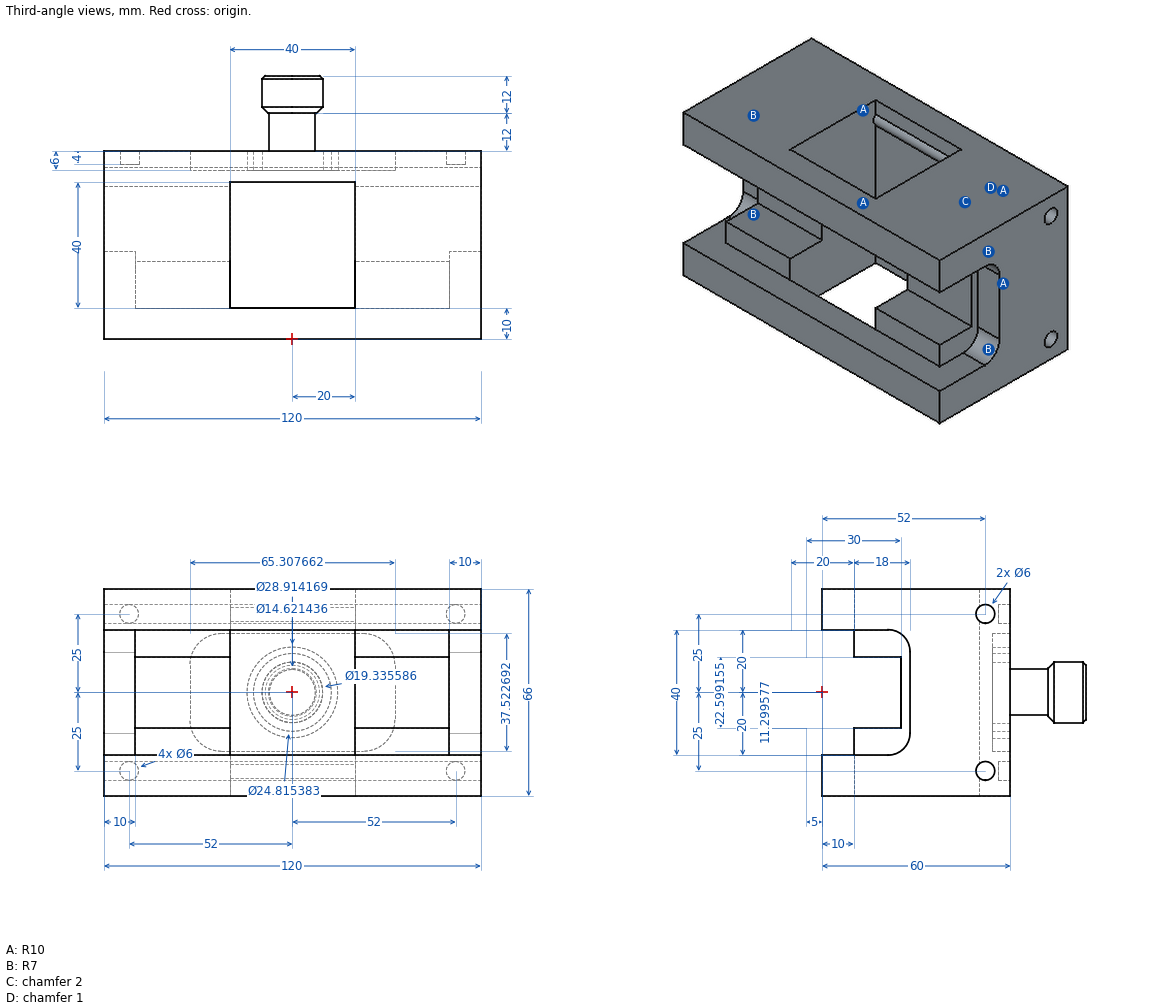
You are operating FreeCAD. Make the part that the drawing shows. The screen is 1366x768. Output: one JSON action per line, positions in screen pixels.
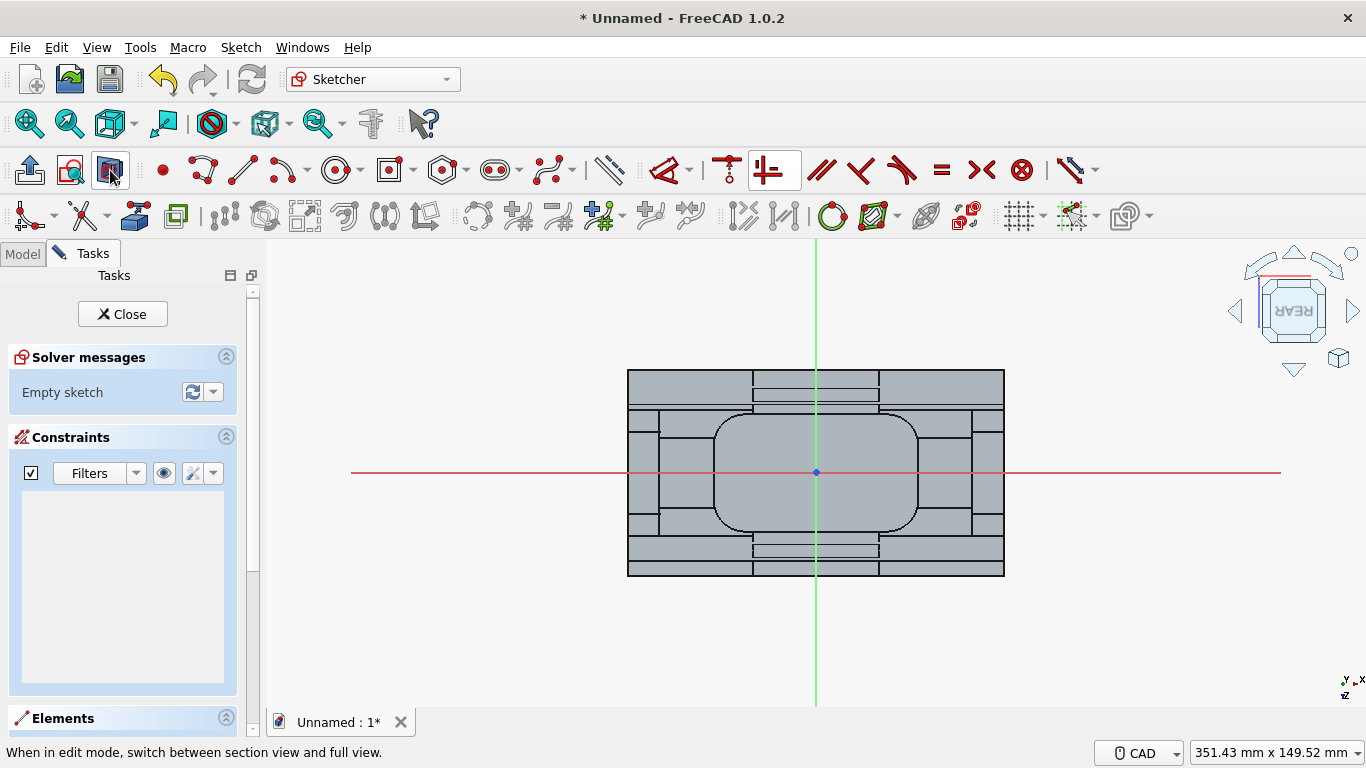
{"action": "scroll", "coordinate": [846, 473], "scroll_direction": "up", "scroll_amount": 6}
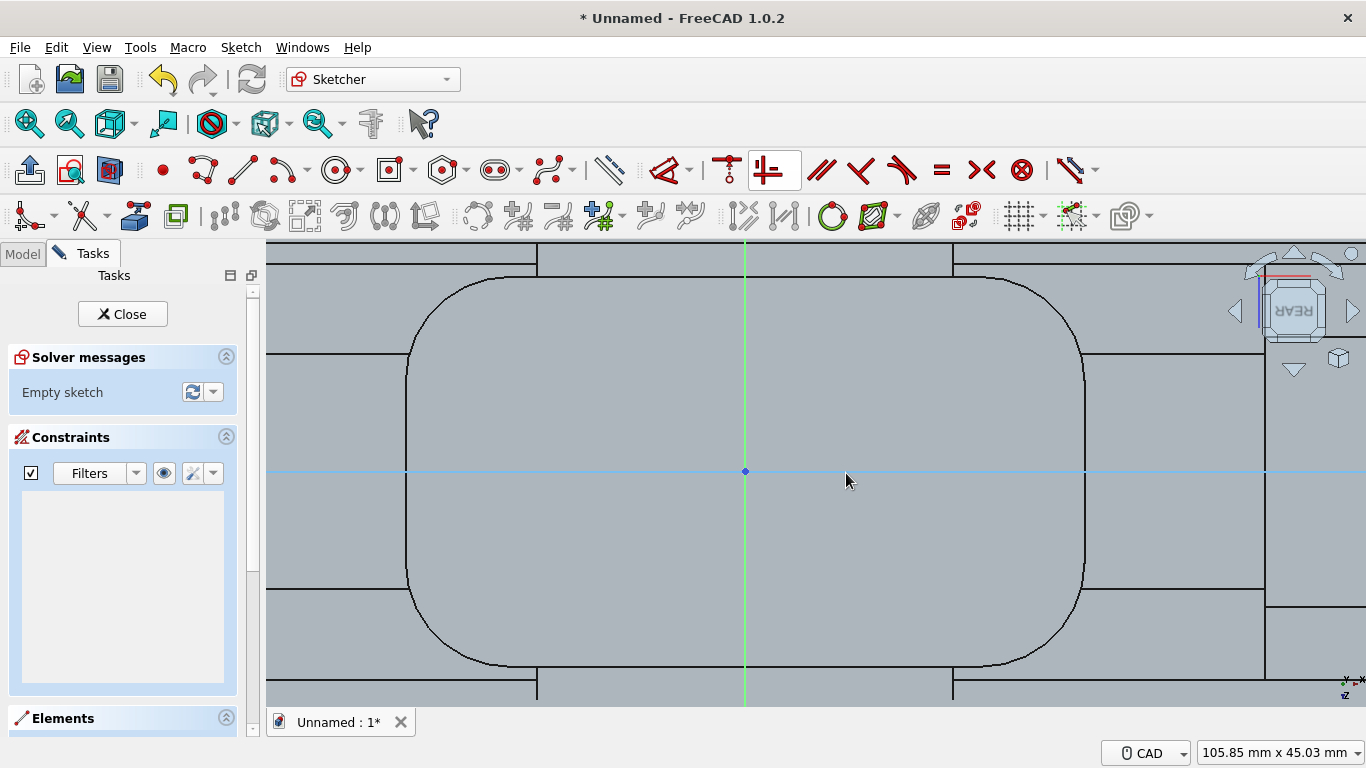
{"action": "left_click", "coordinate": [336, 170]}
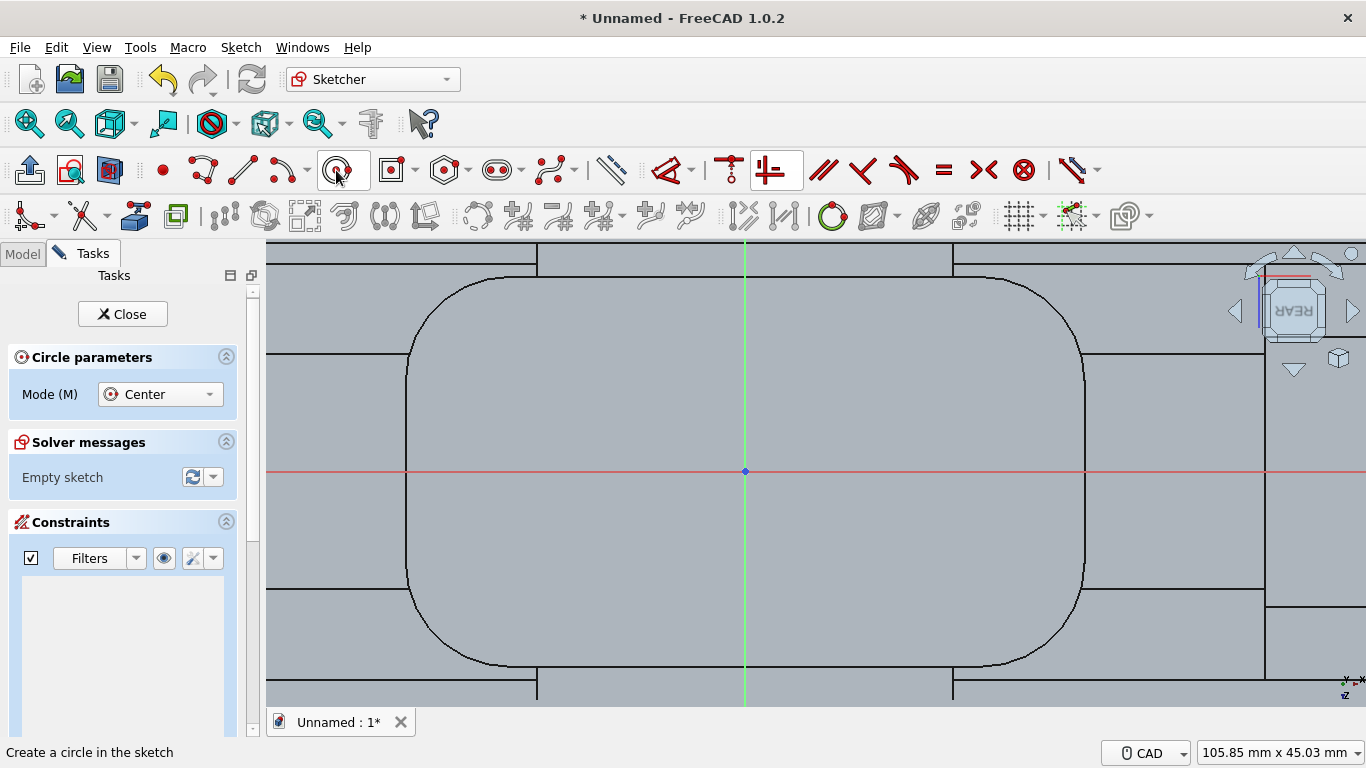
{"action": "left_click", "coordinate": [745, 472]}
{"action": "mouse_move", "coordinate": [851, 366]}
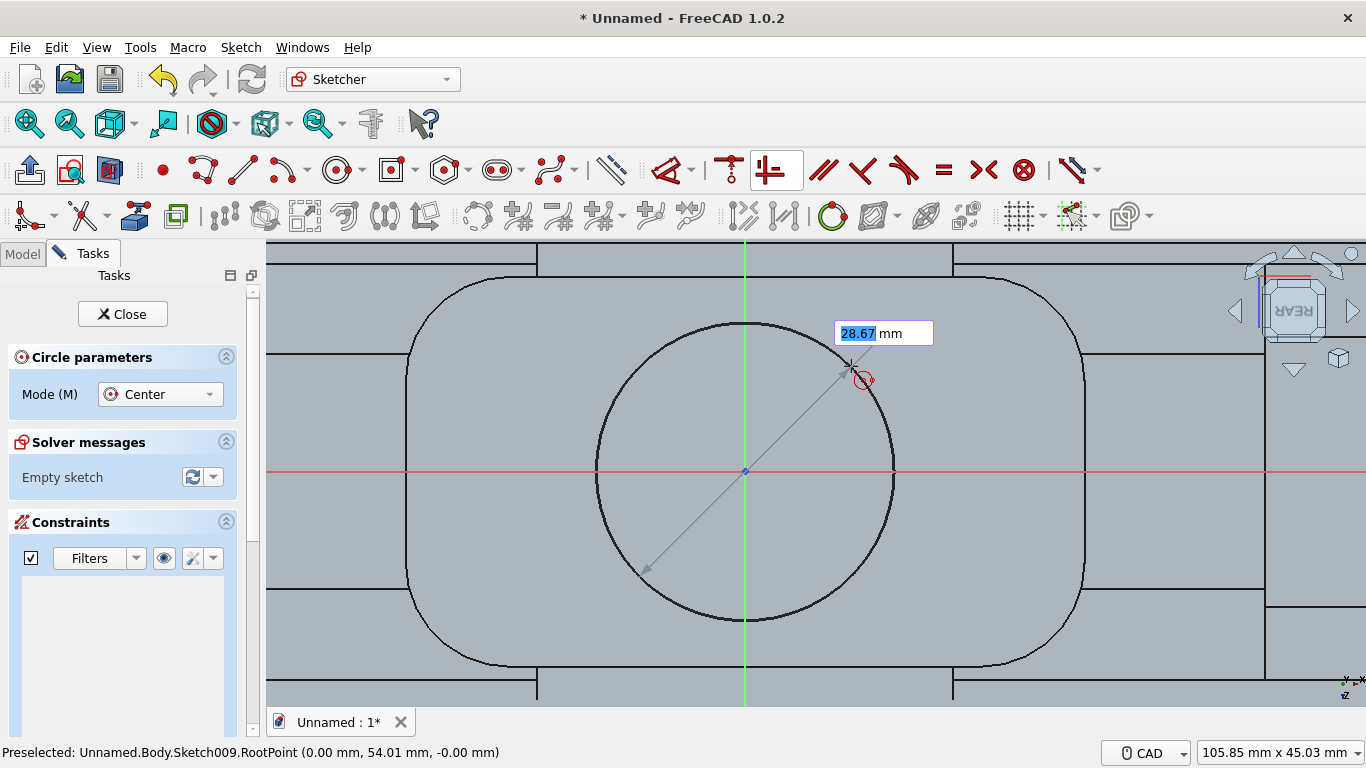
{"action": "type", "text": "28.914169"}
{"action": "key", "text": "Return"}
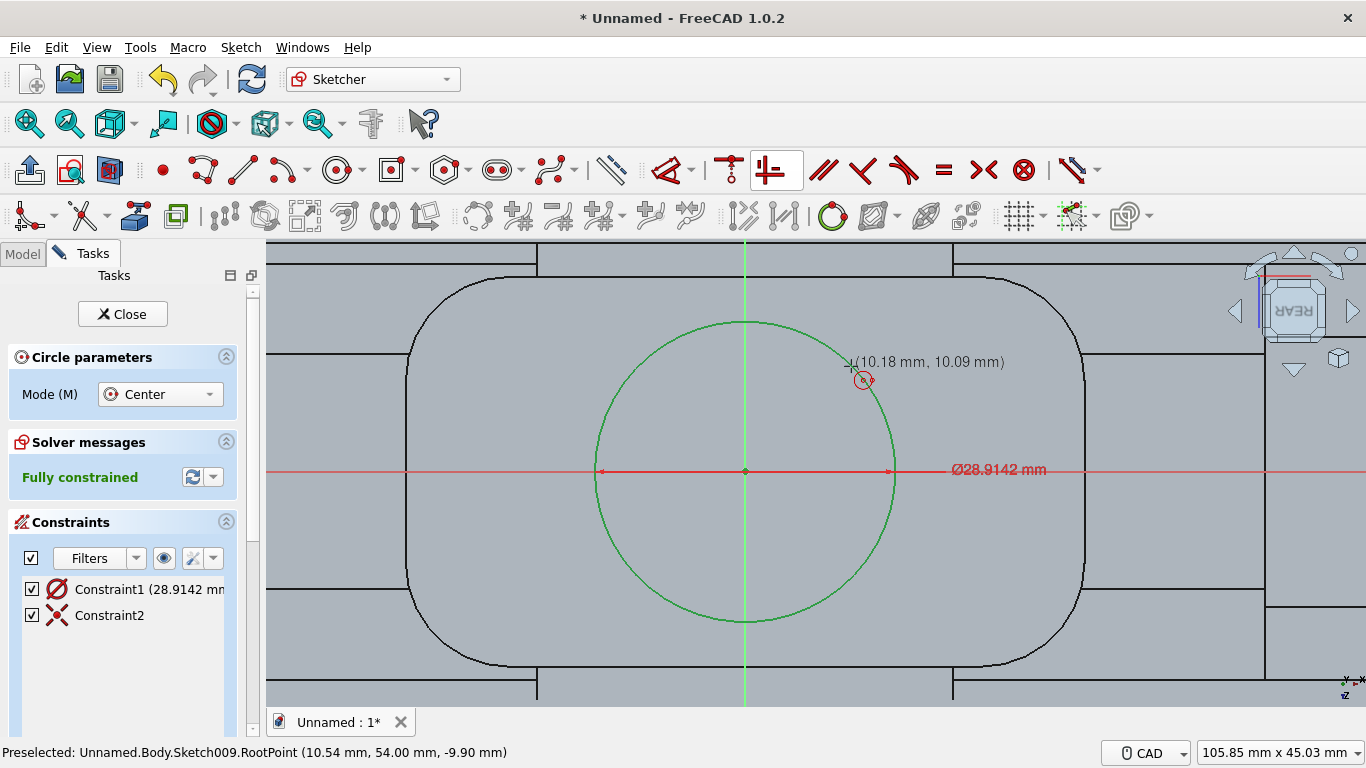
{"action": "left_click", "coordinate": [745, 472]}
{"action": "mouse_move", "coordinate": [836, 381]}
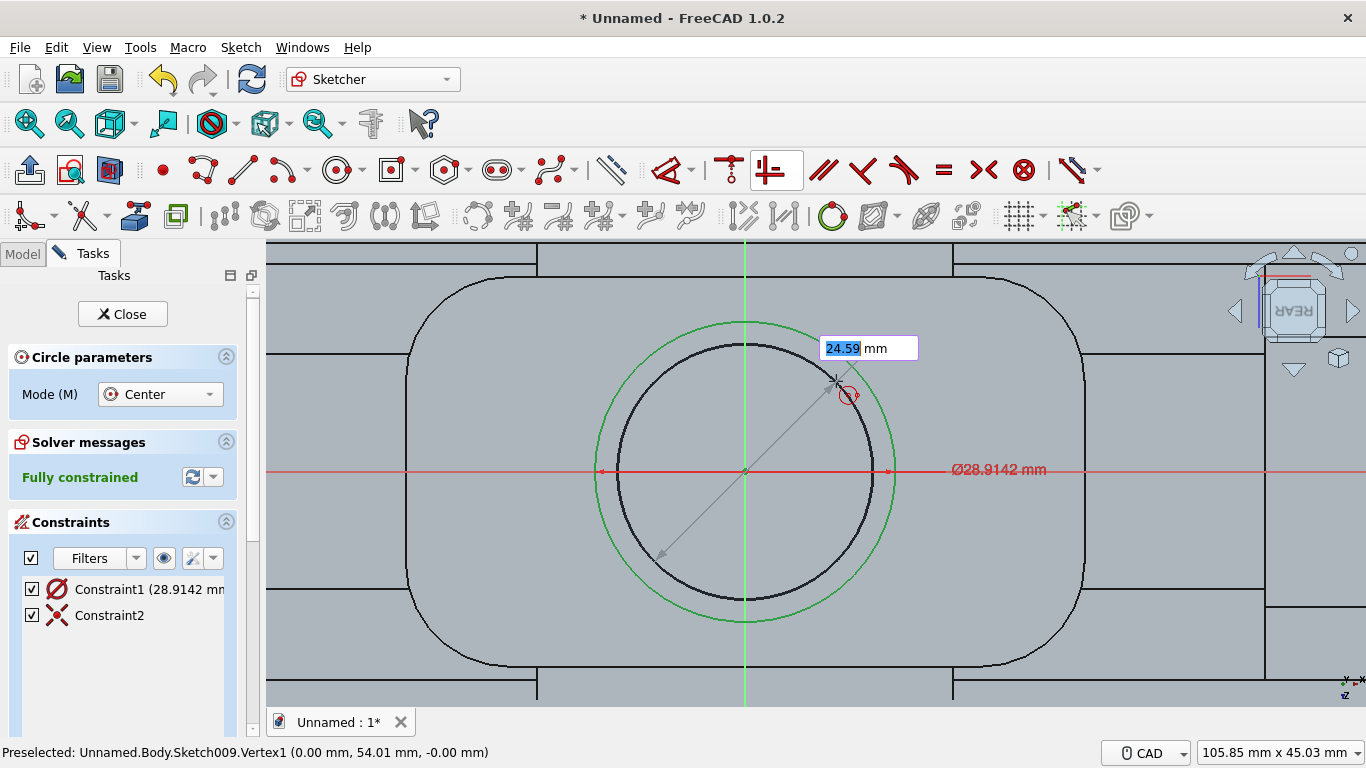
{"action": "type", "text": "24.815383"}
{"action": "key", "text": "Return"}
{"action": "key", "text": "Escape"}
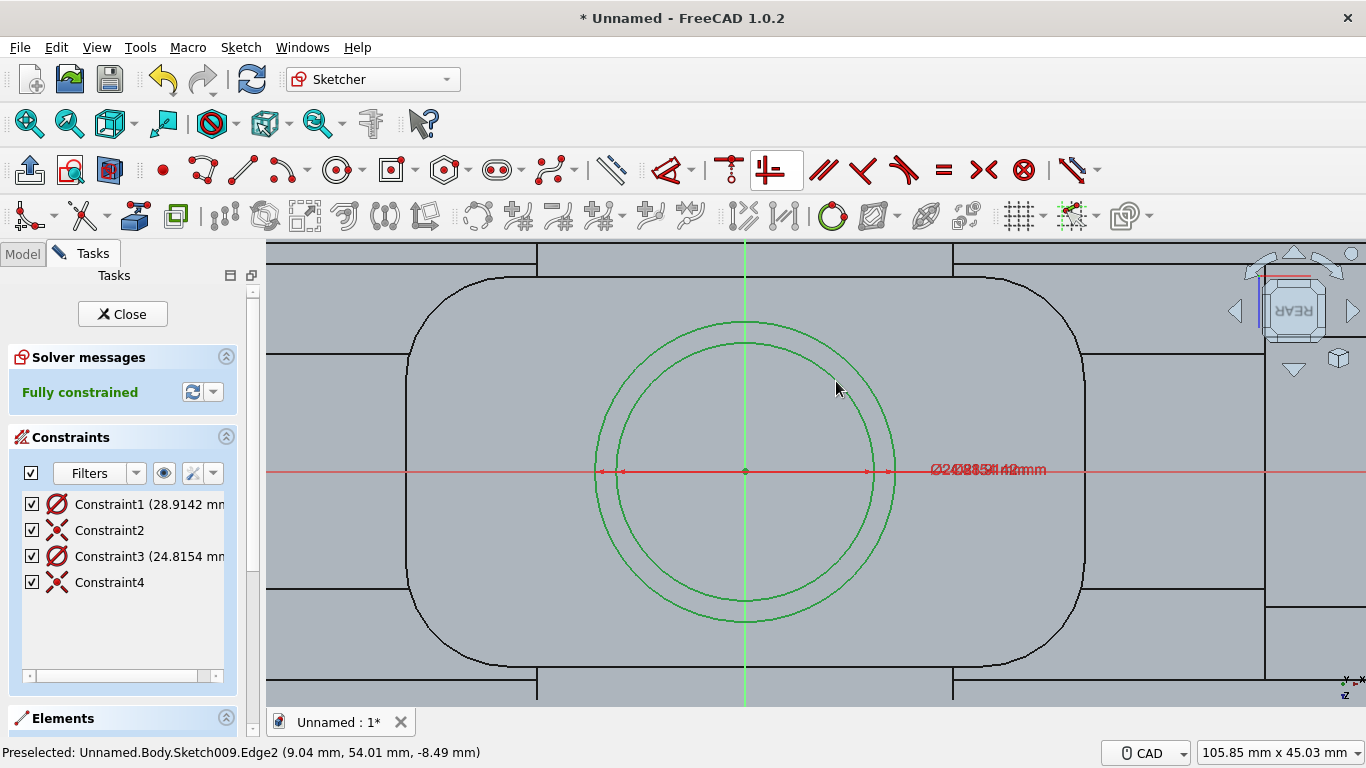
{"action": "left_click", "coordinate": [123, 314]}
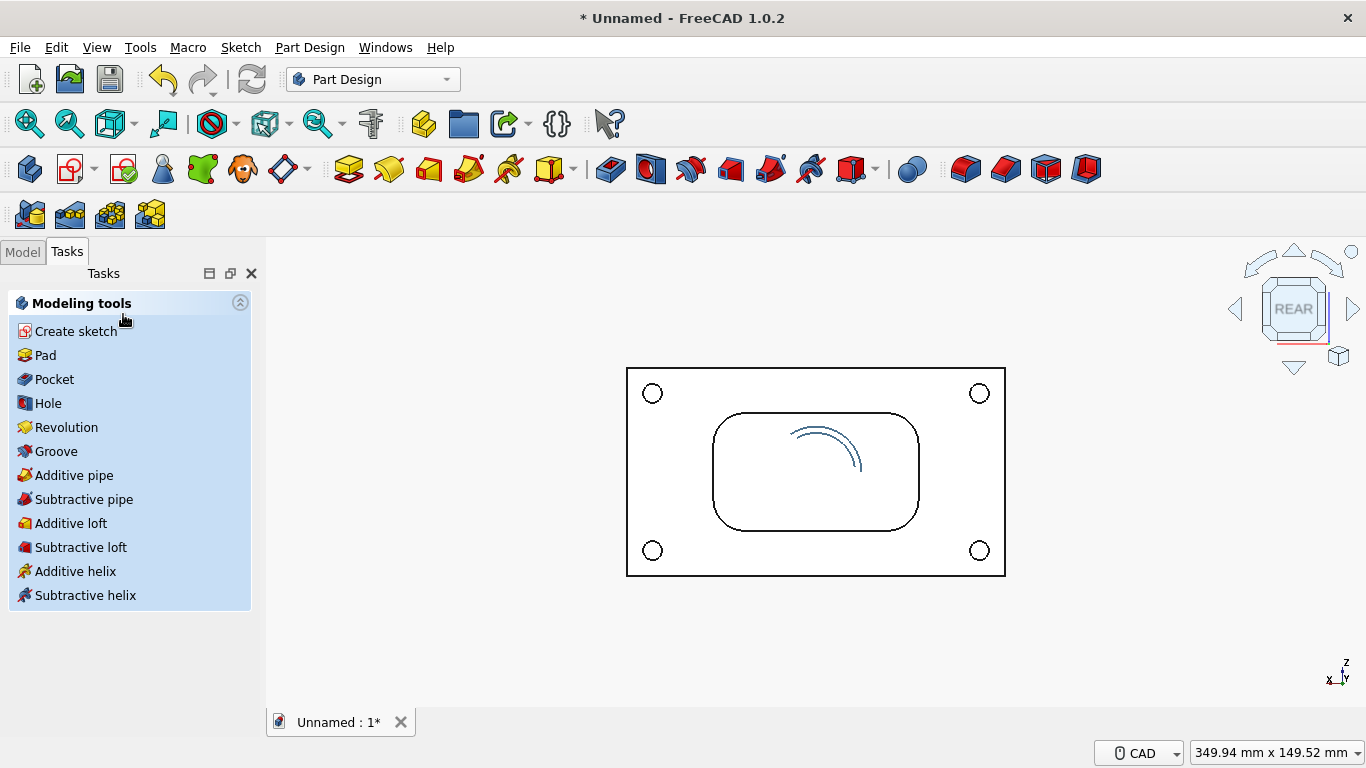
{"action": "left_click", "coordinate": [350, 170]}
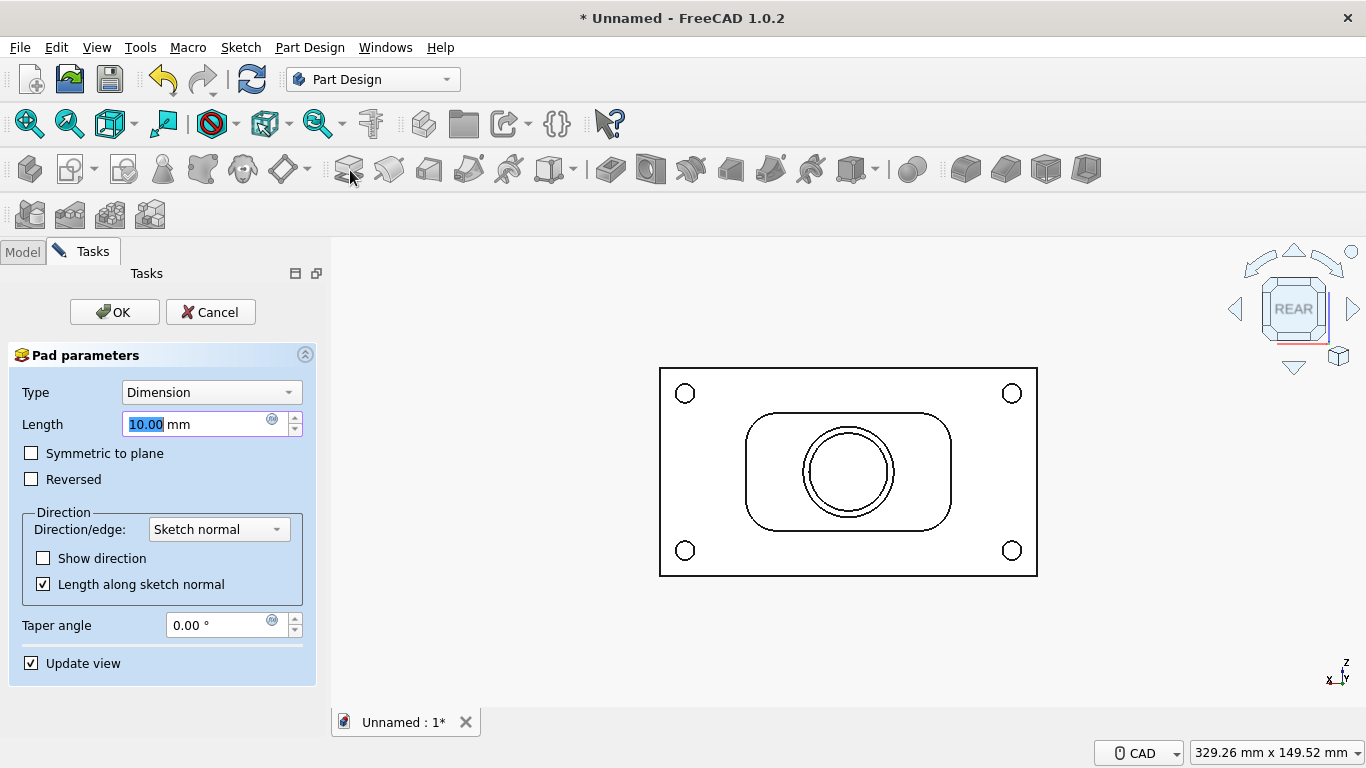
{"action": "type", "text": "6"}
{"action": "key", "text": "Tab"}